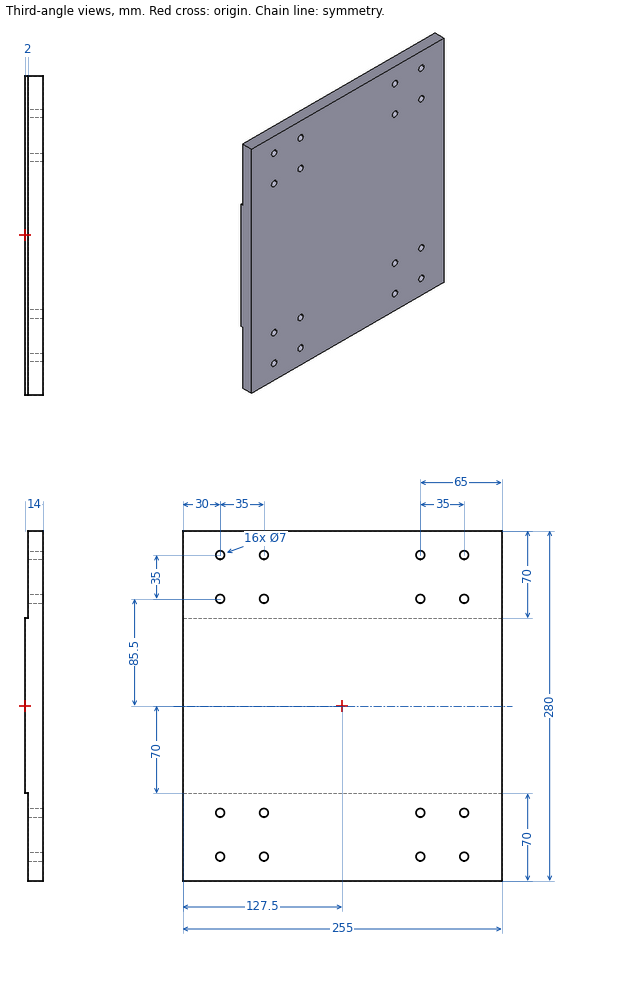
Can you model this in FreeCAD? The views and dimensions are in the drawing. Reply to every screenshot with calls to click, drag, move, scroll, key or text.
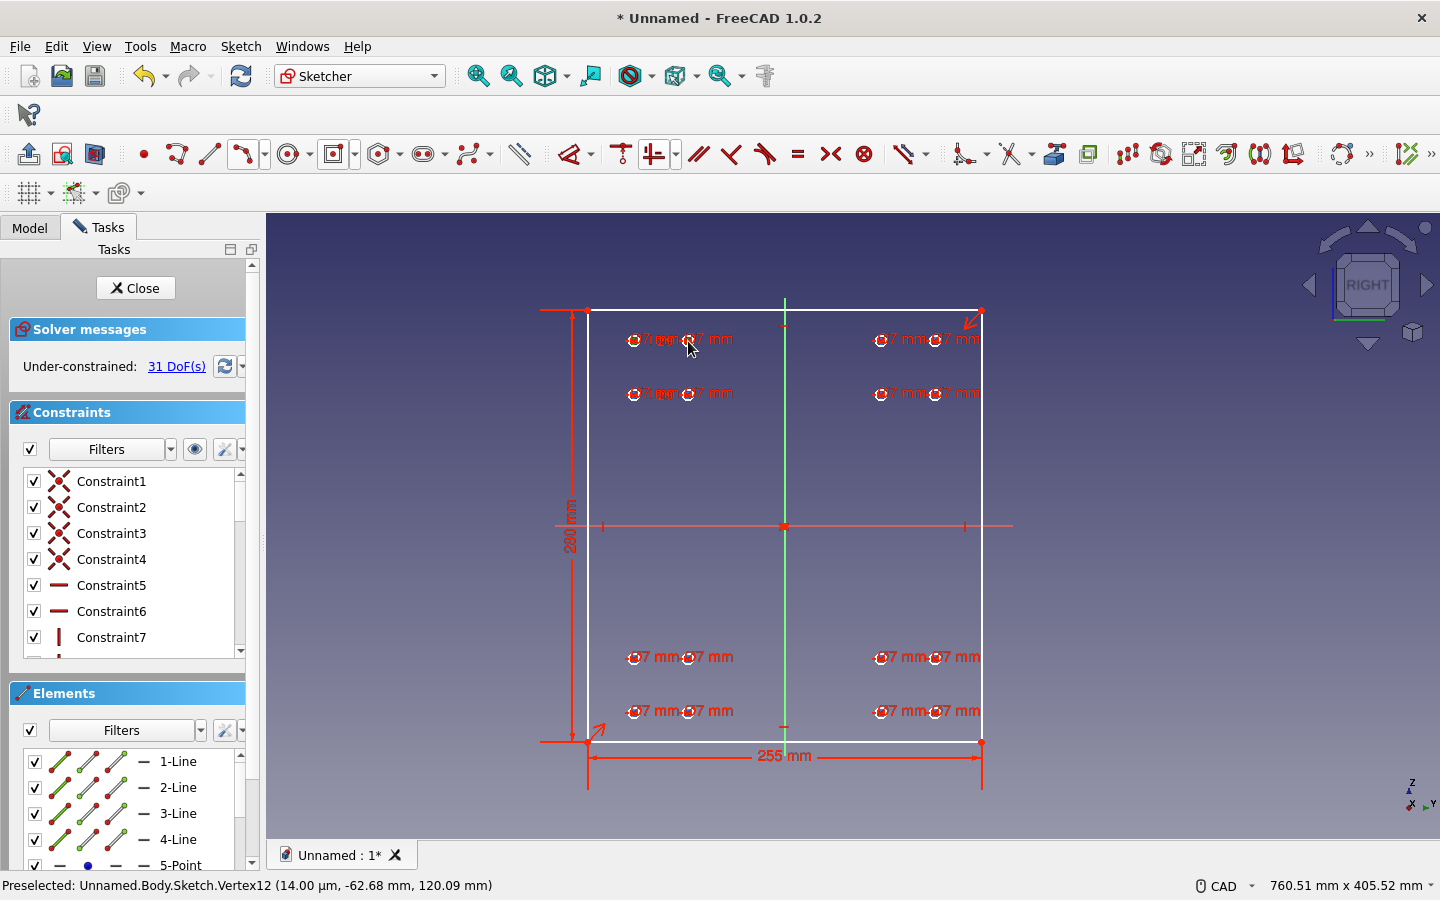
click(676, 154)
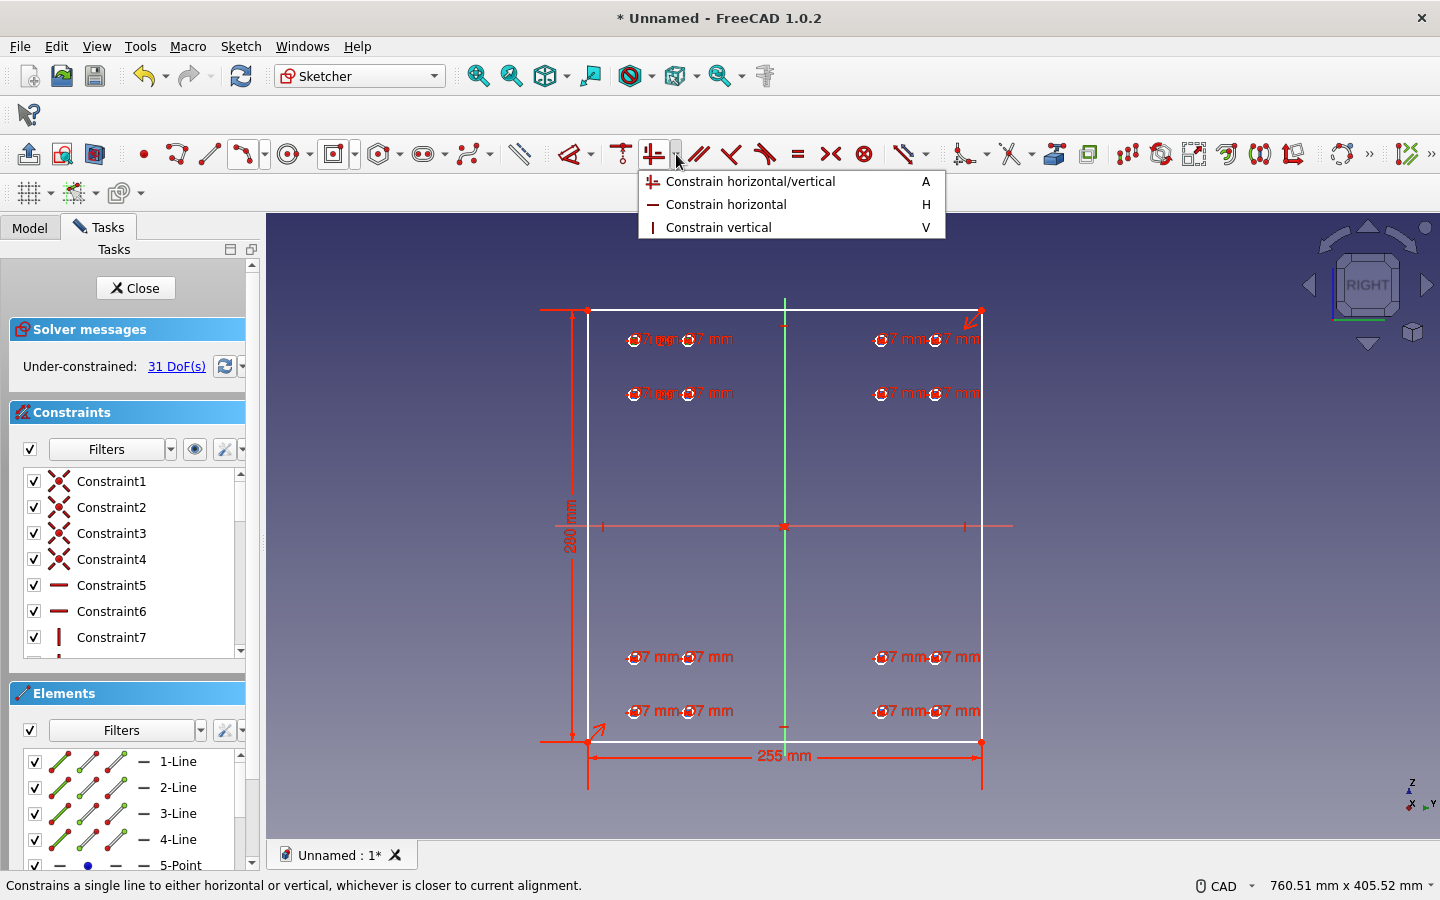
click(792, 204)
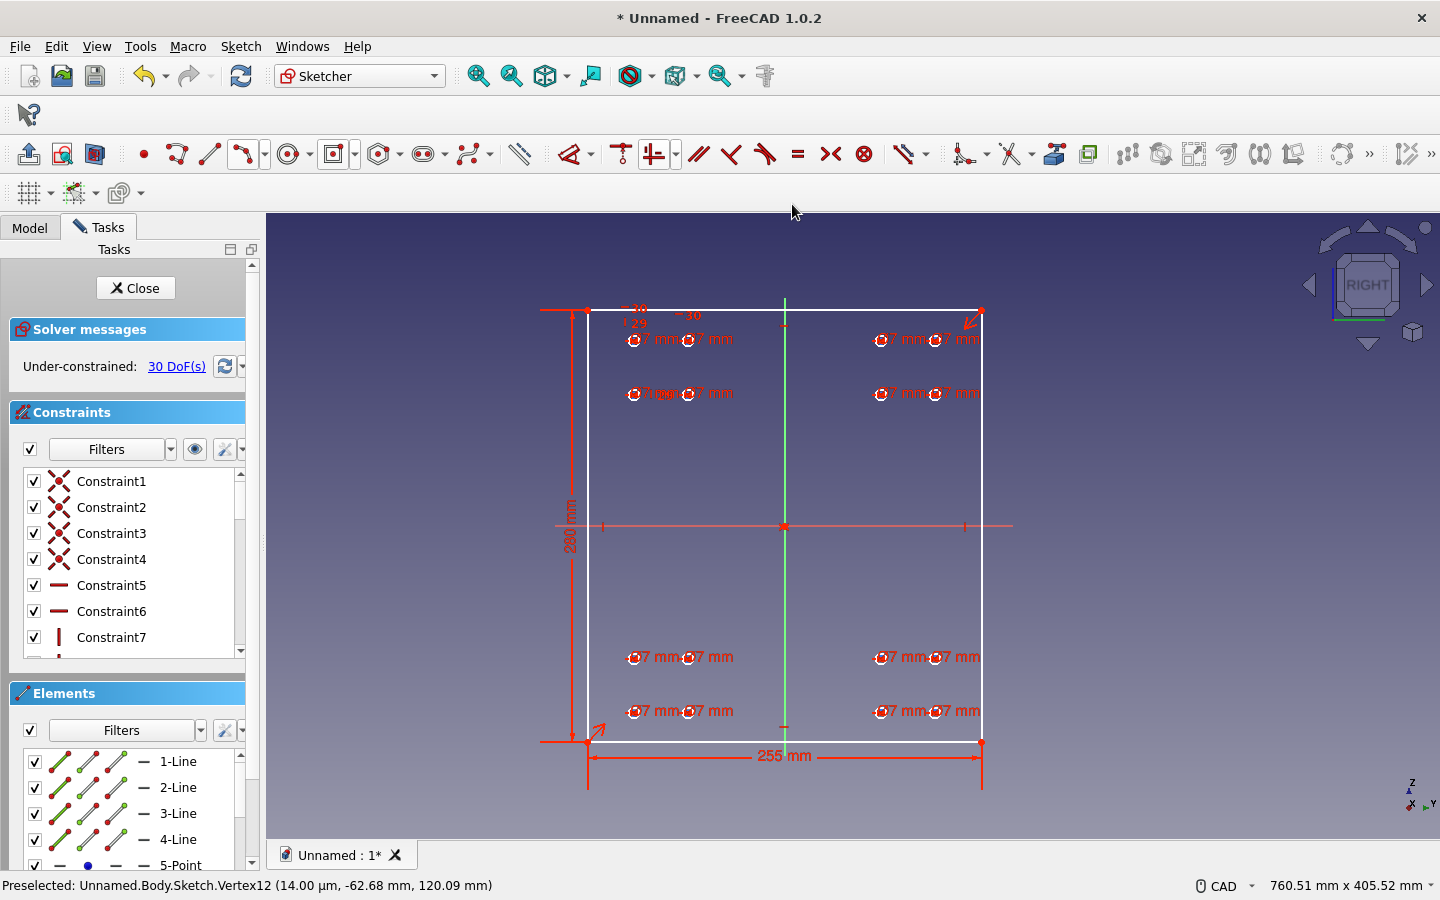
click(688, 341)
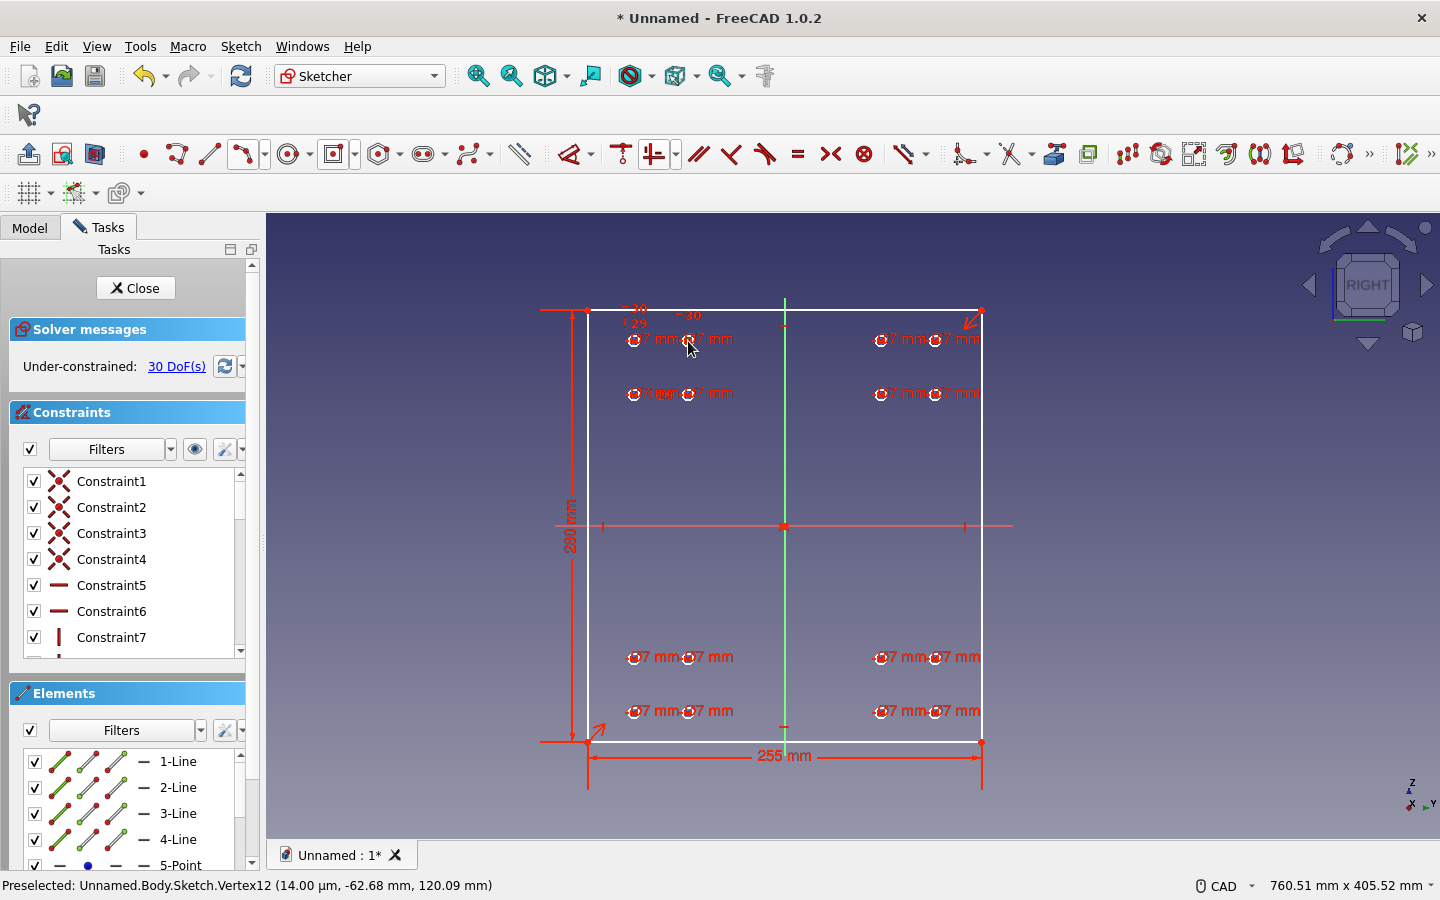
click(688, 395)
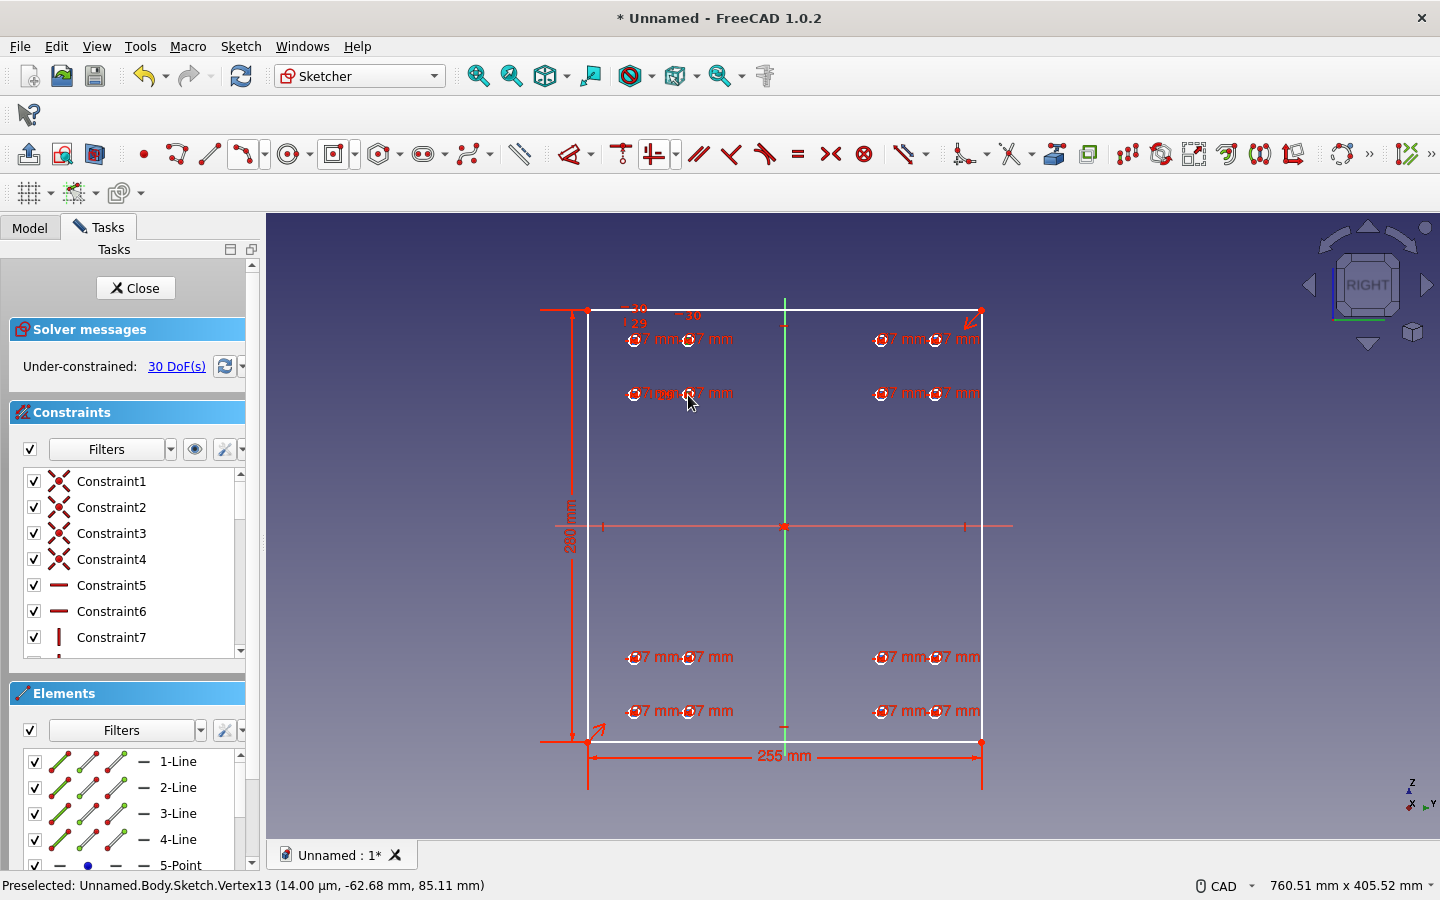
key(v)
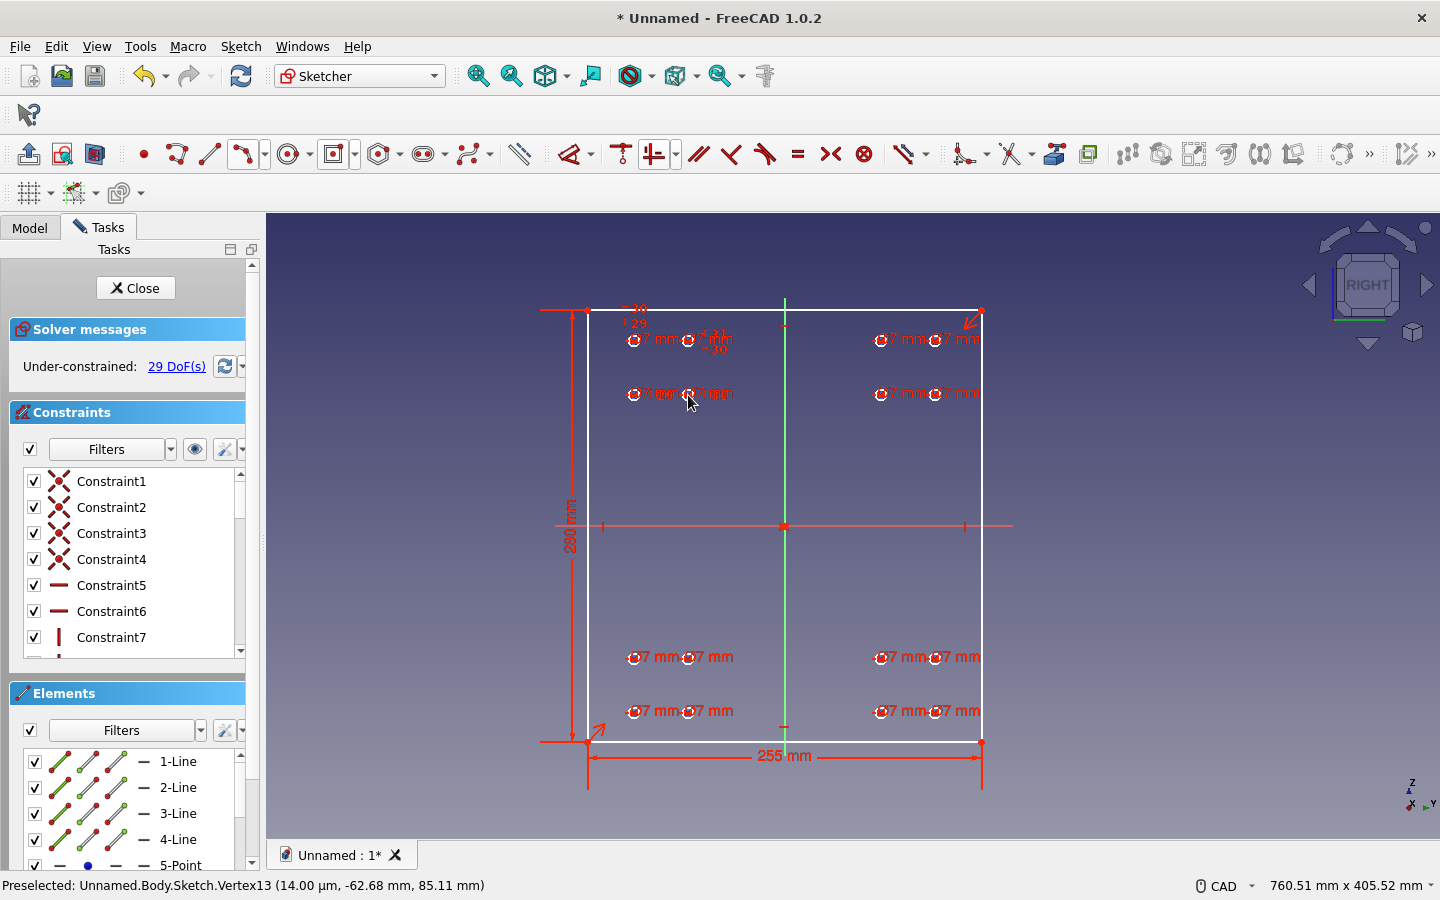
click(634, 395)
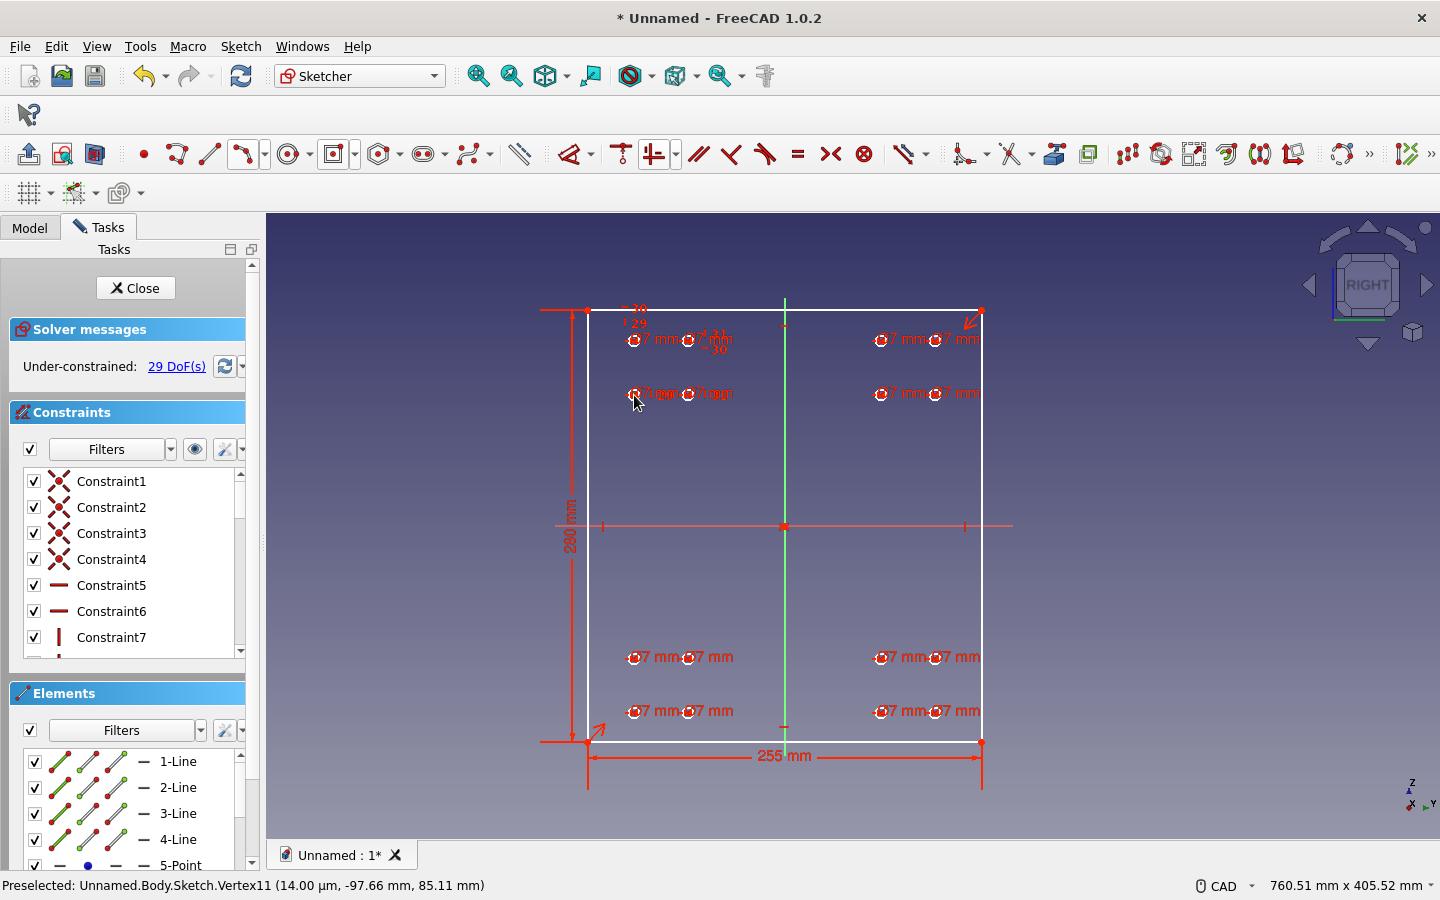
click(688, 395)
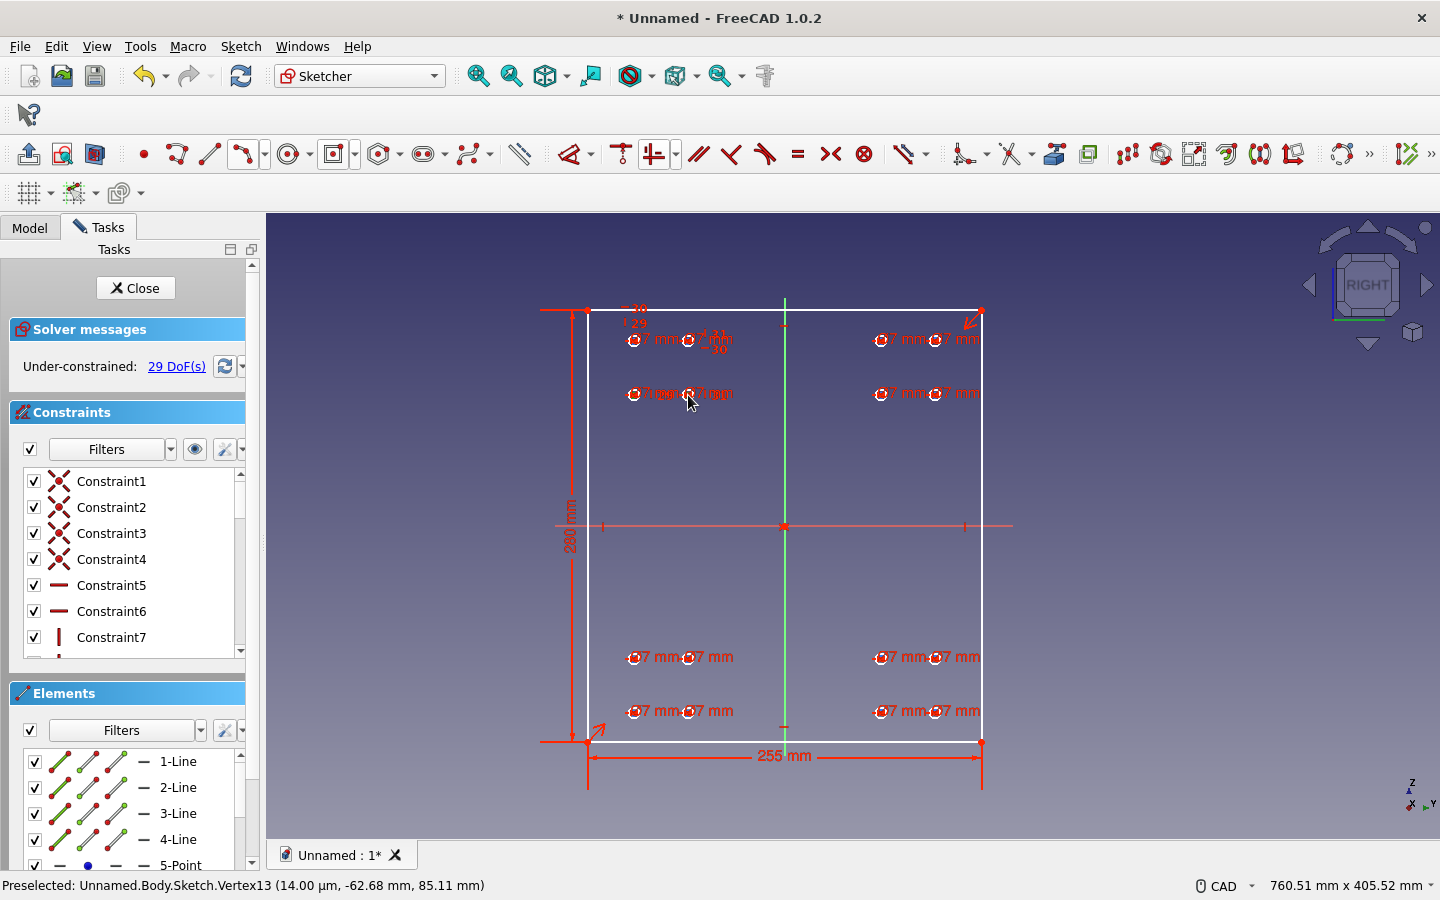
click(676, 154)